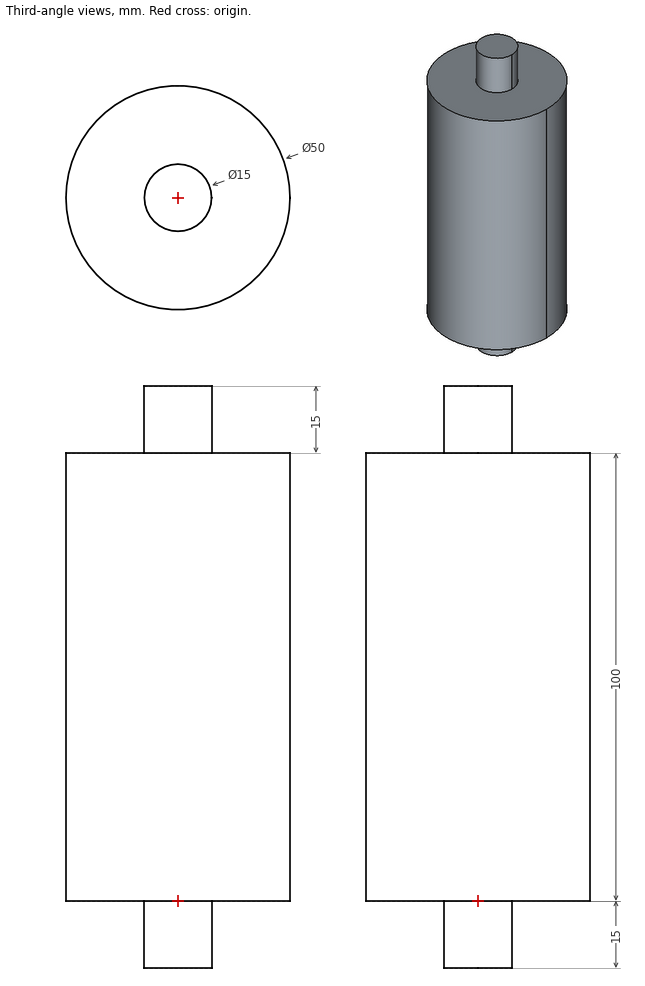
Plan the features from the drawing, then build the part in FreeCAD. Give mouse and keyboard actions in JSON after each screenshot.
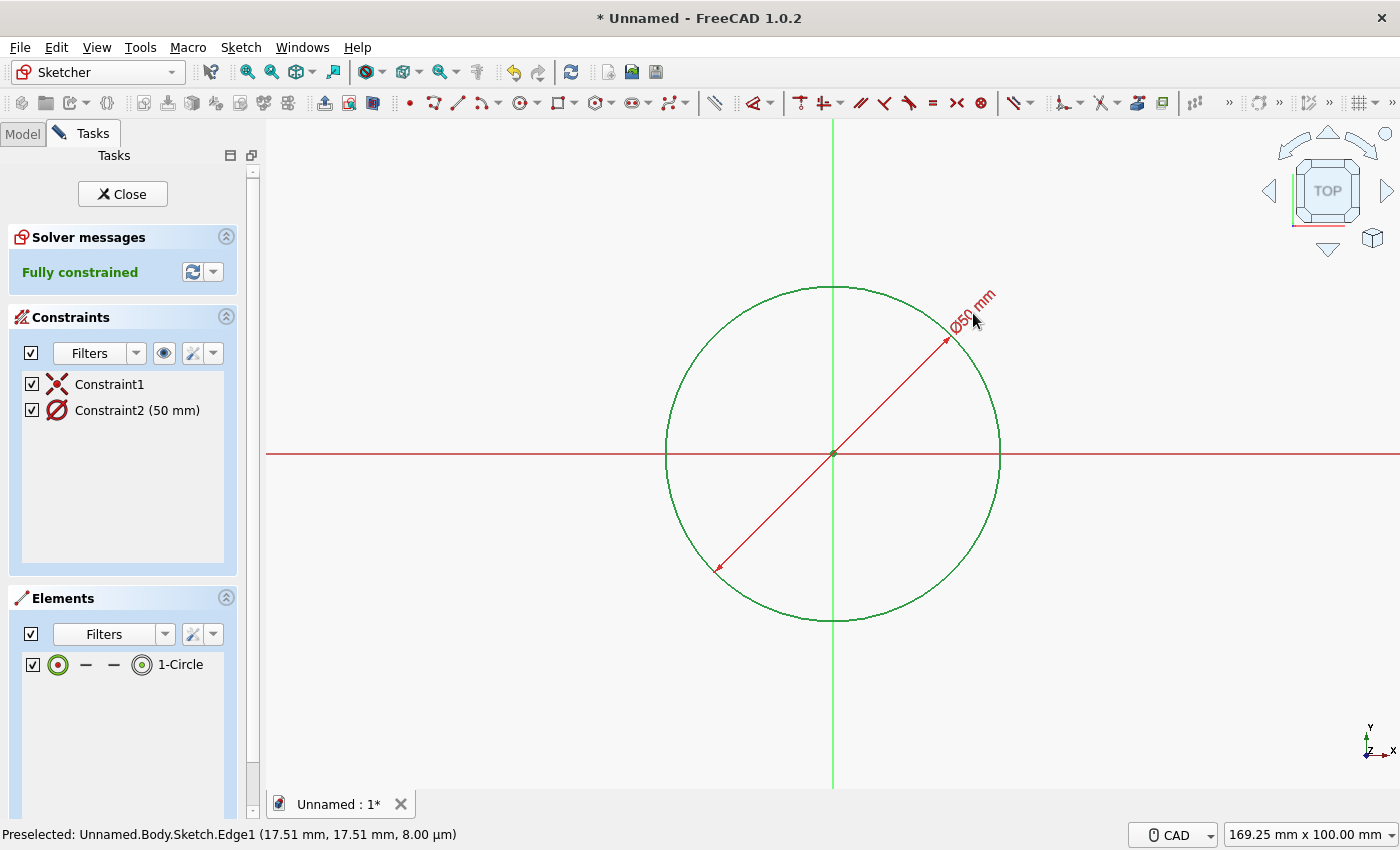
{"action": "left_click", "coordinate": [123, 194]}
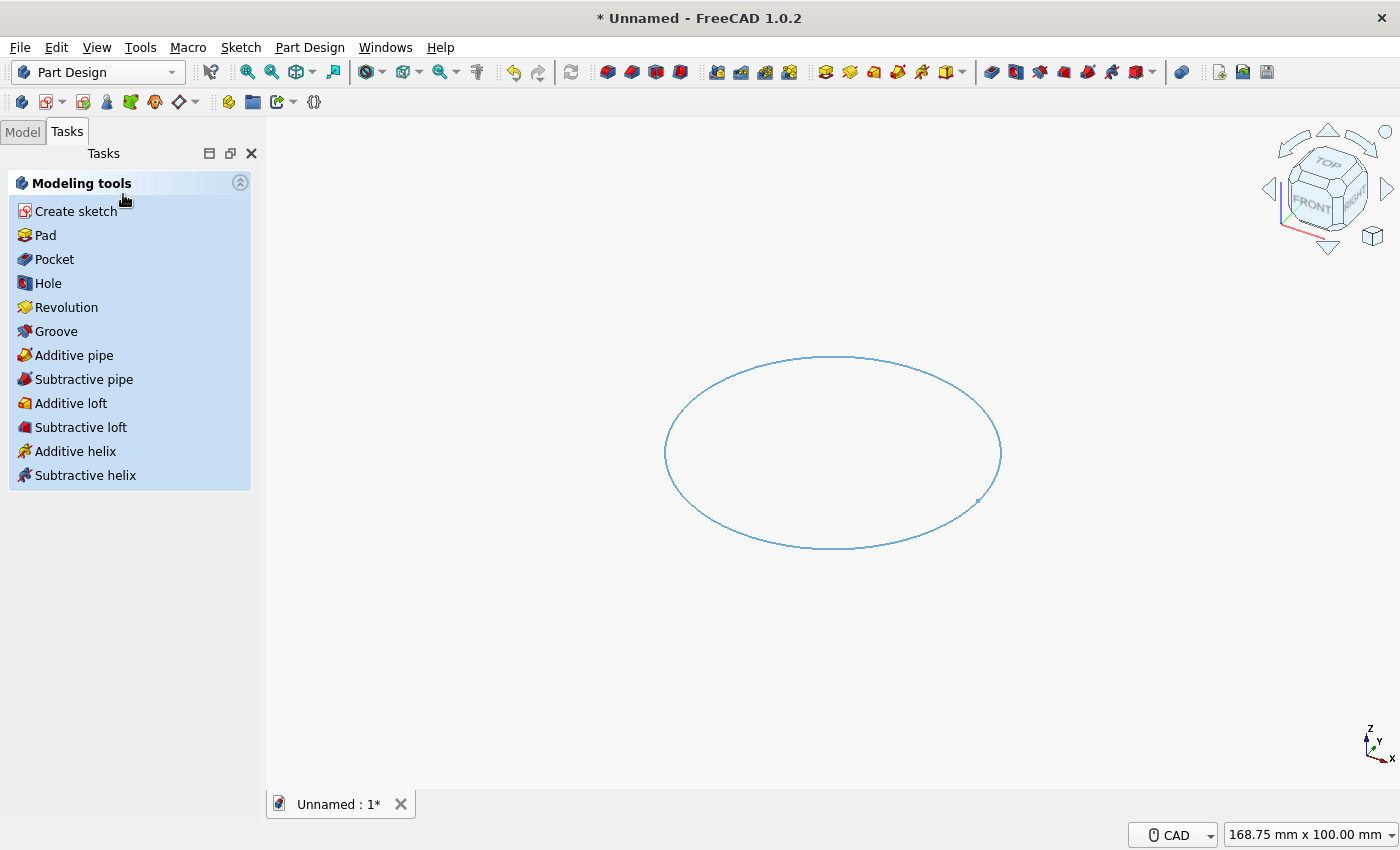
{"action": "left_click", "coordinate": [826, 72]}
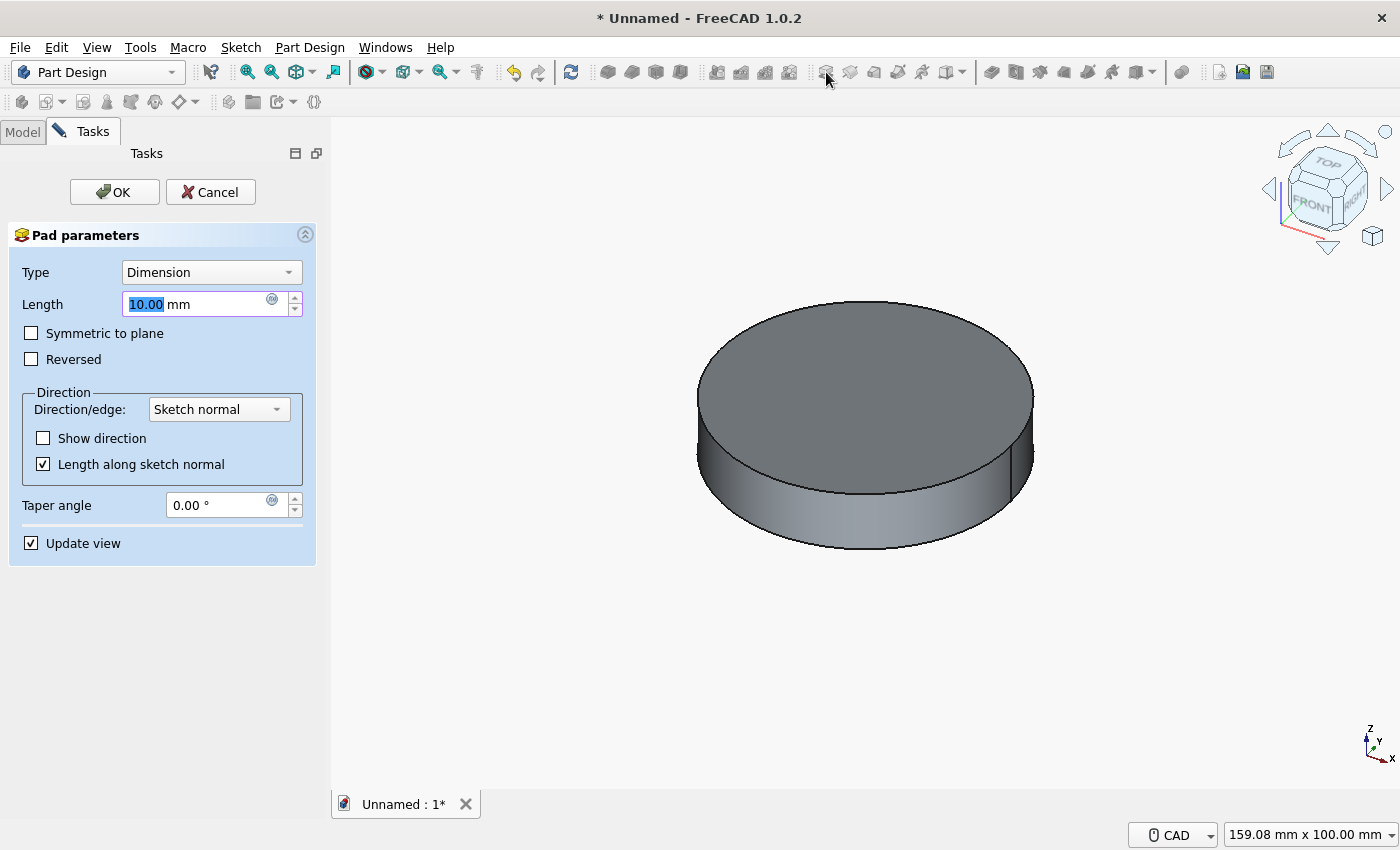
{"action": "type", "text": "100"}
{"action": "key", "text": "Tab"}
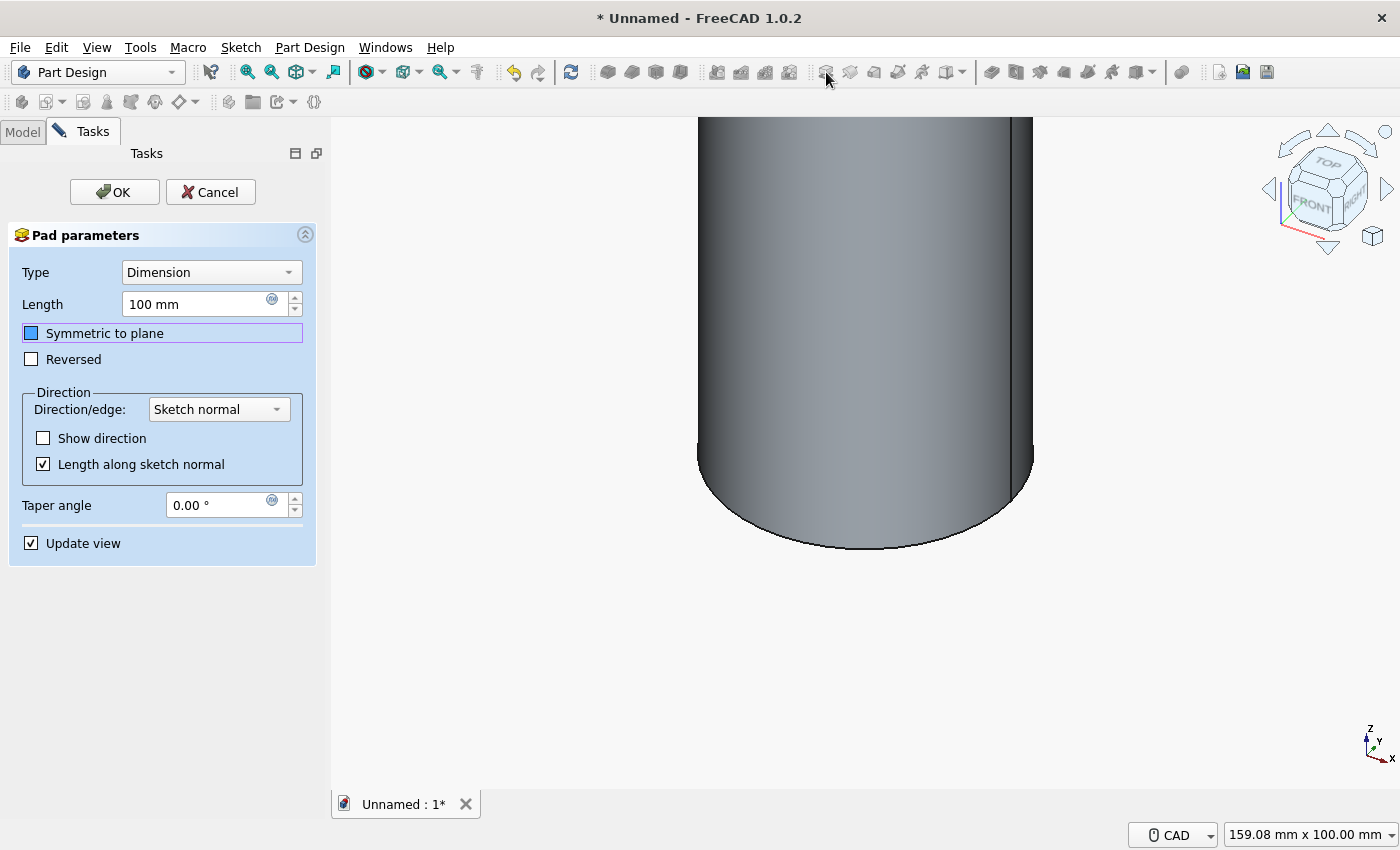
{"action": "left_click", "coordinate": [115, 192]}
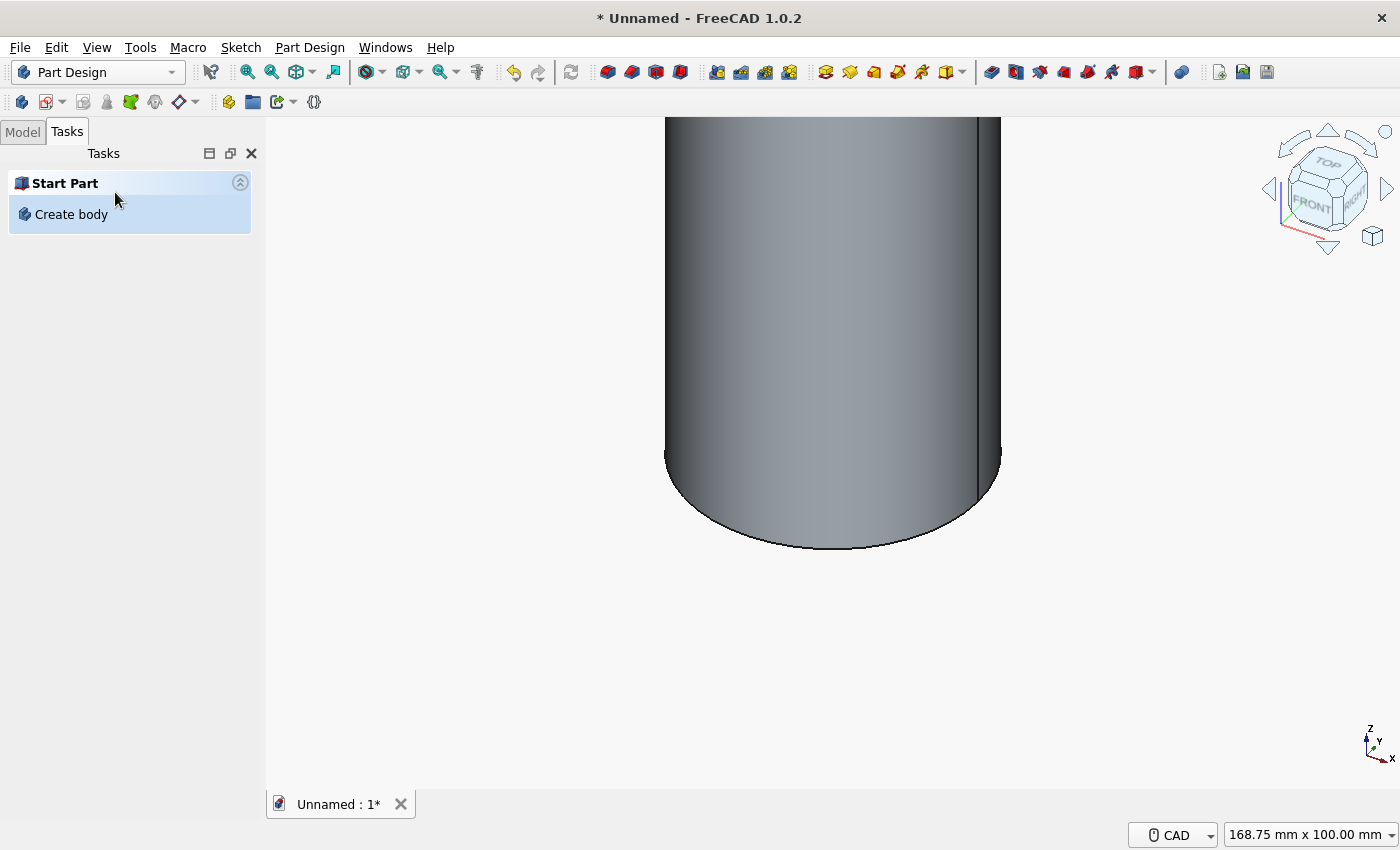
{"action": "left_click", "coordinate": [248, 72]}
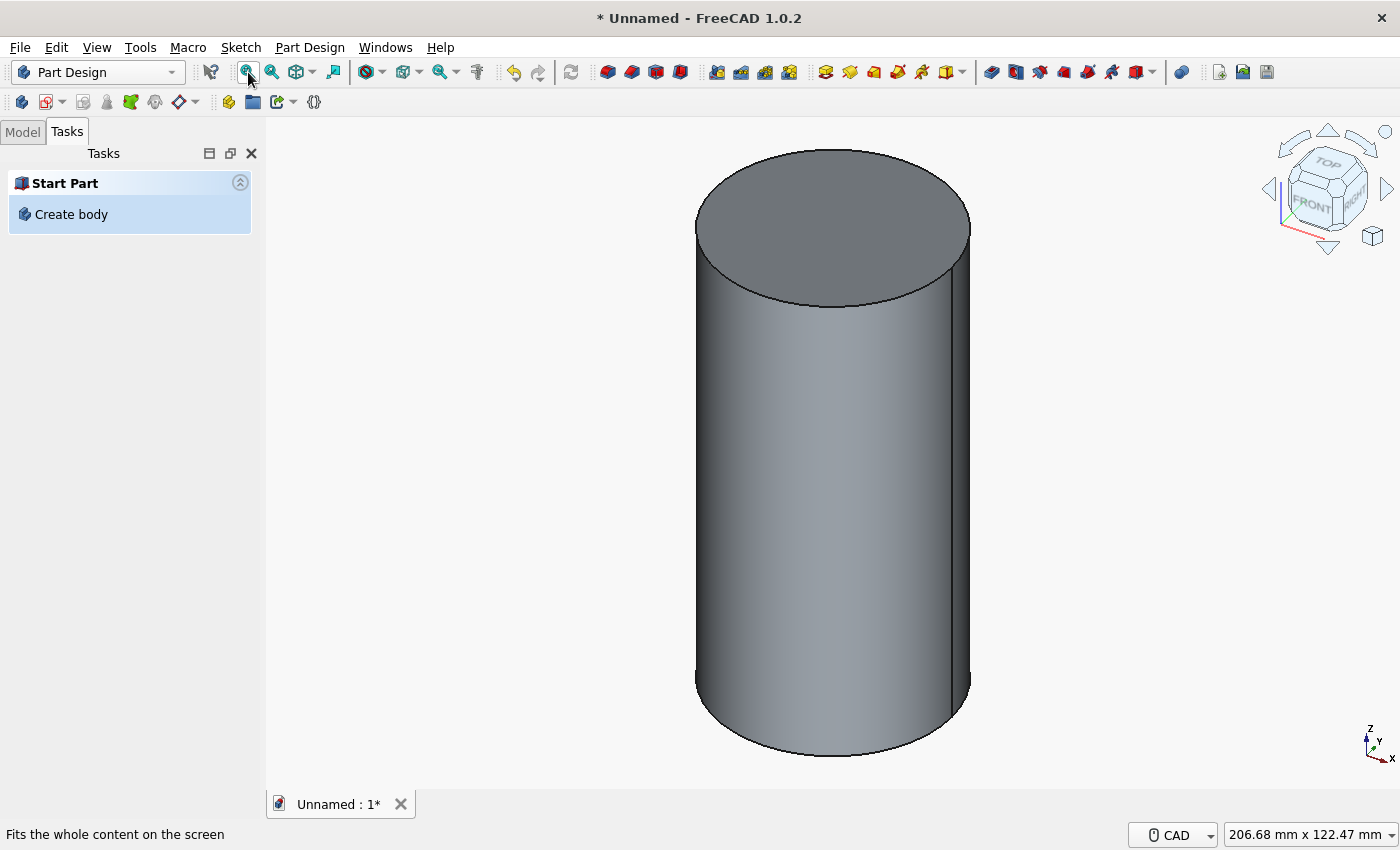
{"action": "left_click", "coordinate": [833, 227]}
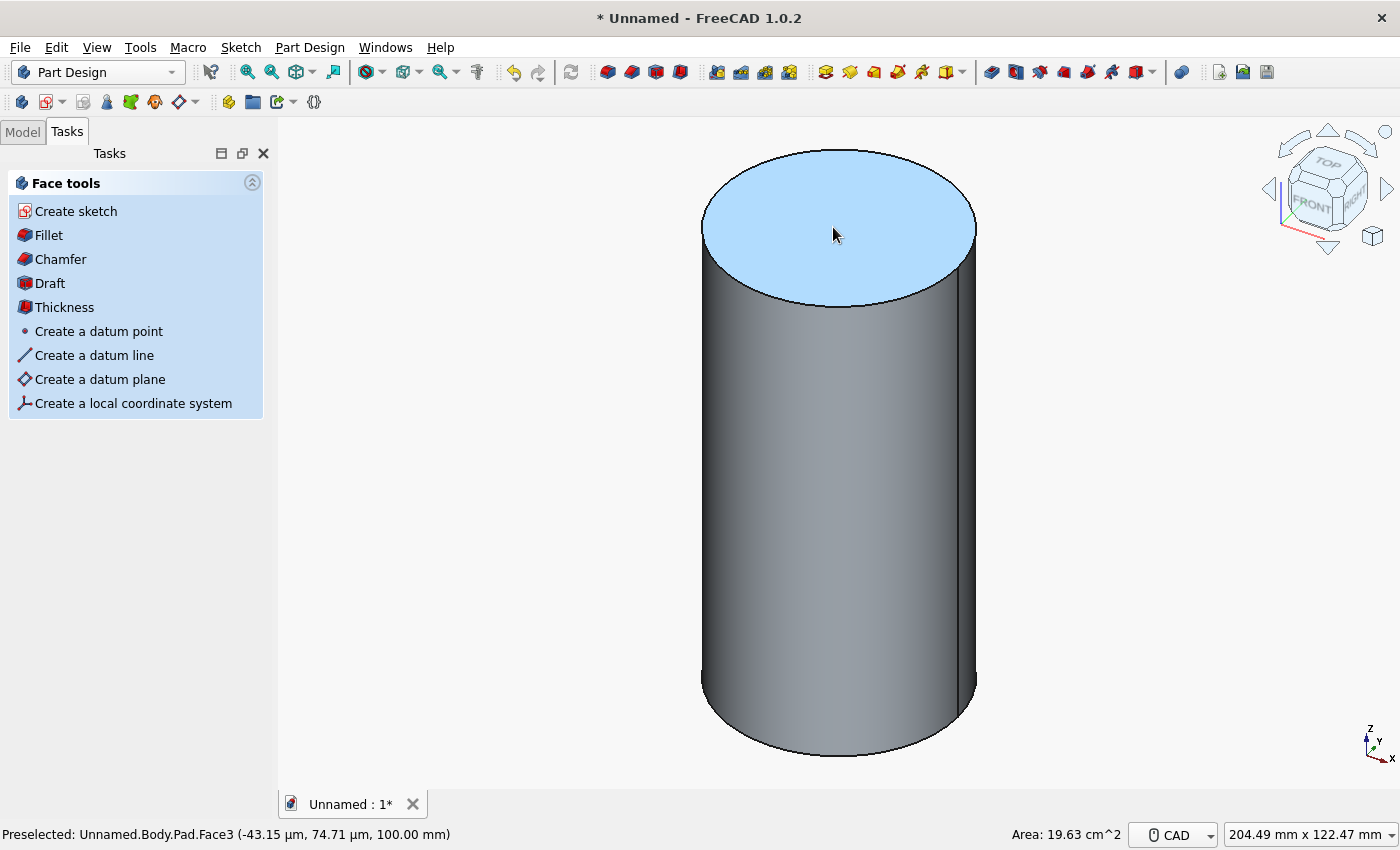
{"action": "left_click", "coordinate": [46, 102]}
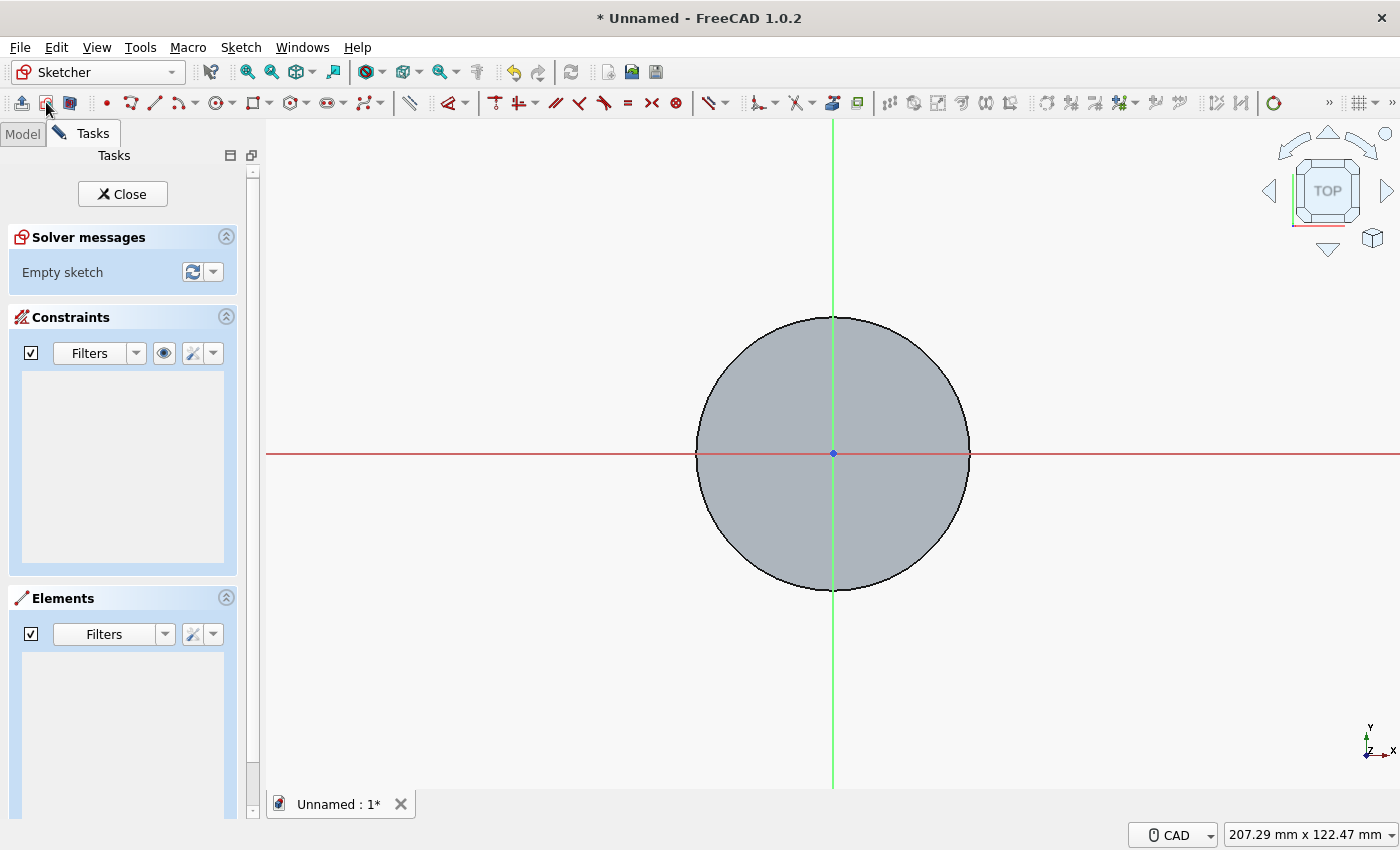
{"action": "scroll", "coordinate": [850, 454], "scroll_direction": "up", "scroll_amount": 8}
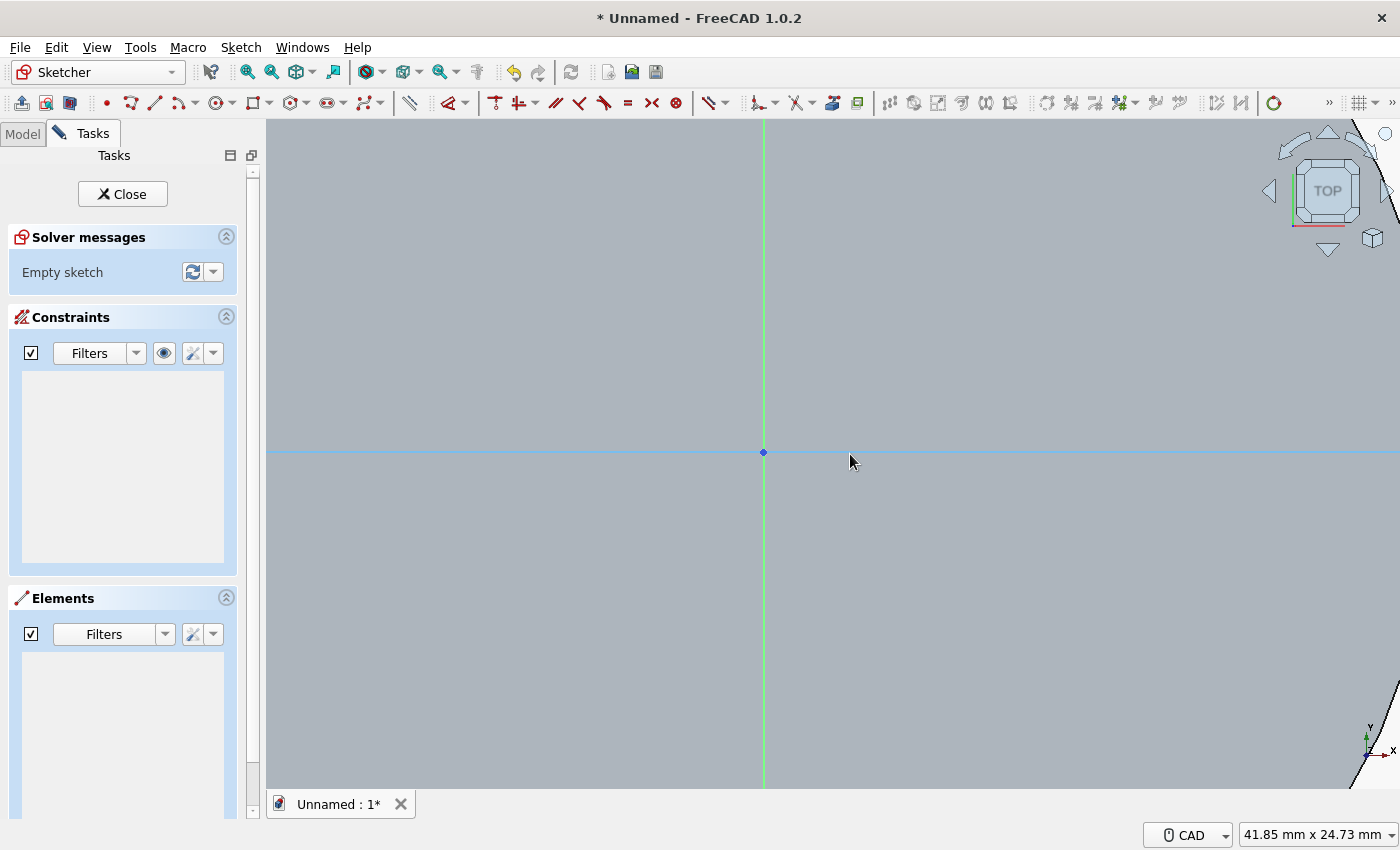
{"action": "key", "text": "g c"}